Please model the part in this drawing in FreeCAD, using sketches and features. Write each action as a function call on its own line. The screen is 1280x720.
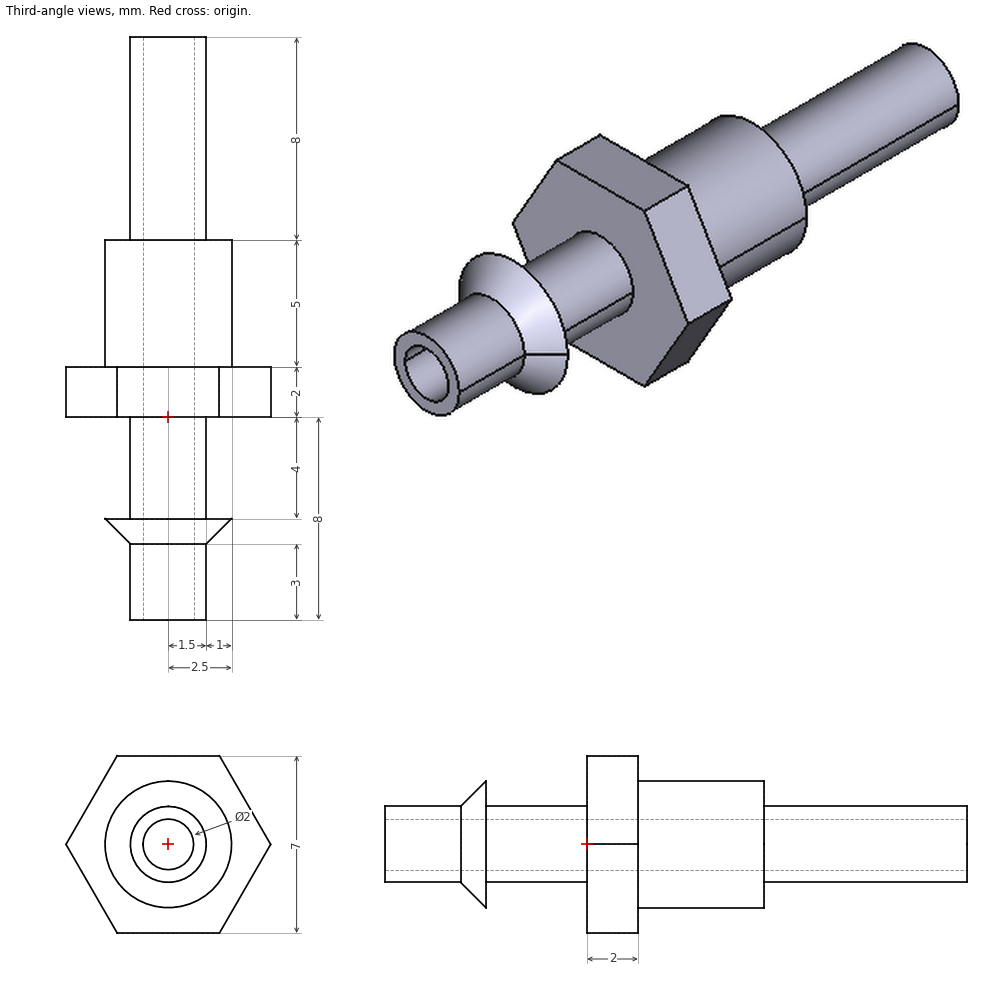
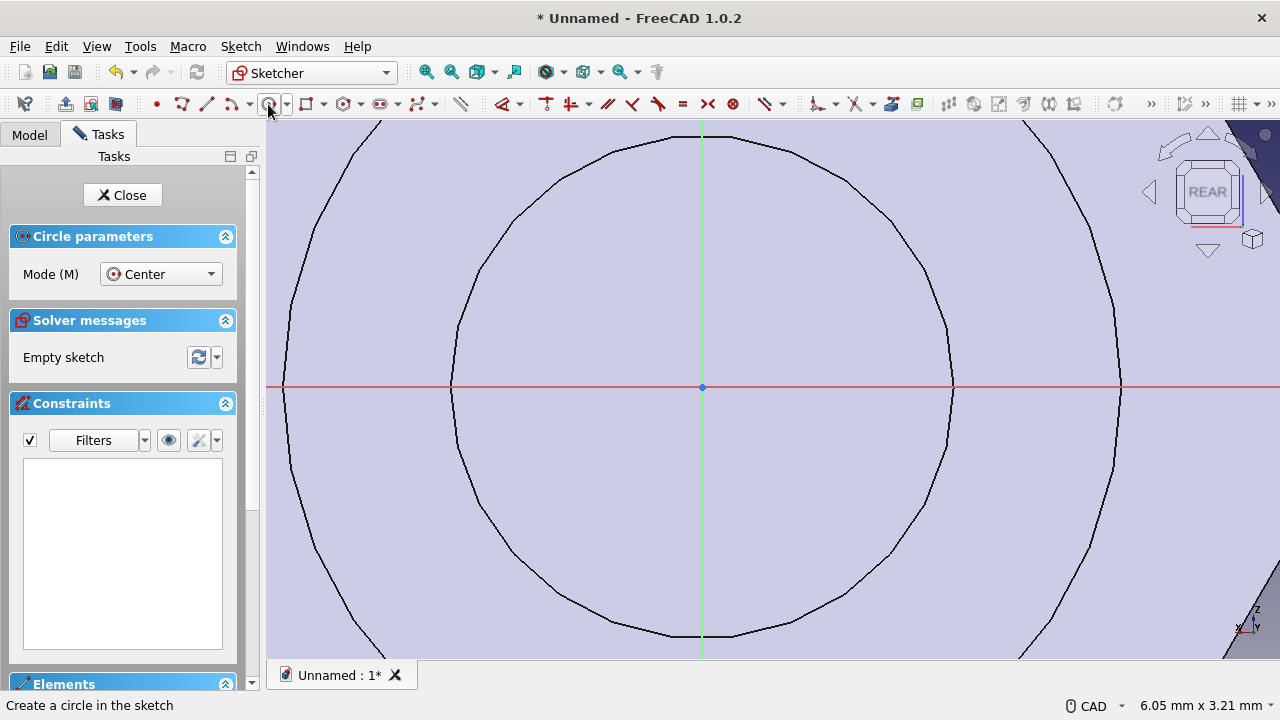
click(702, 387)
move(821, 269)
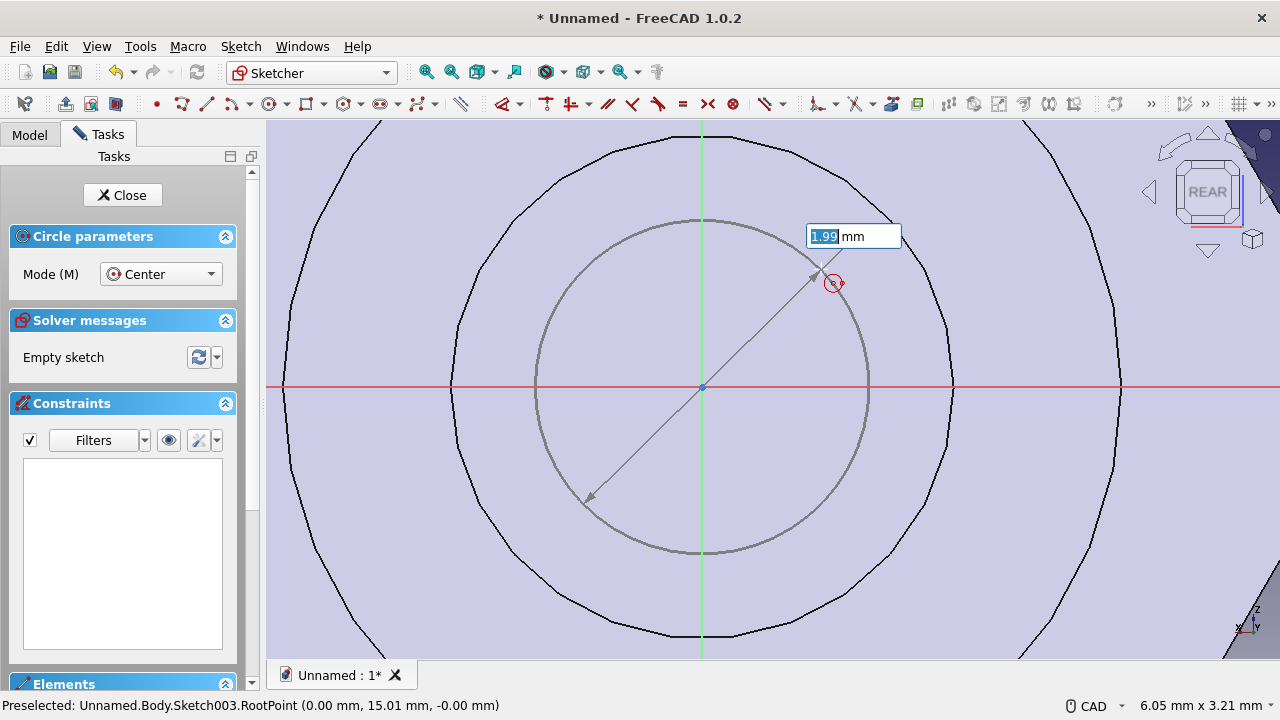
text(2)
key(Return)
key(Escape)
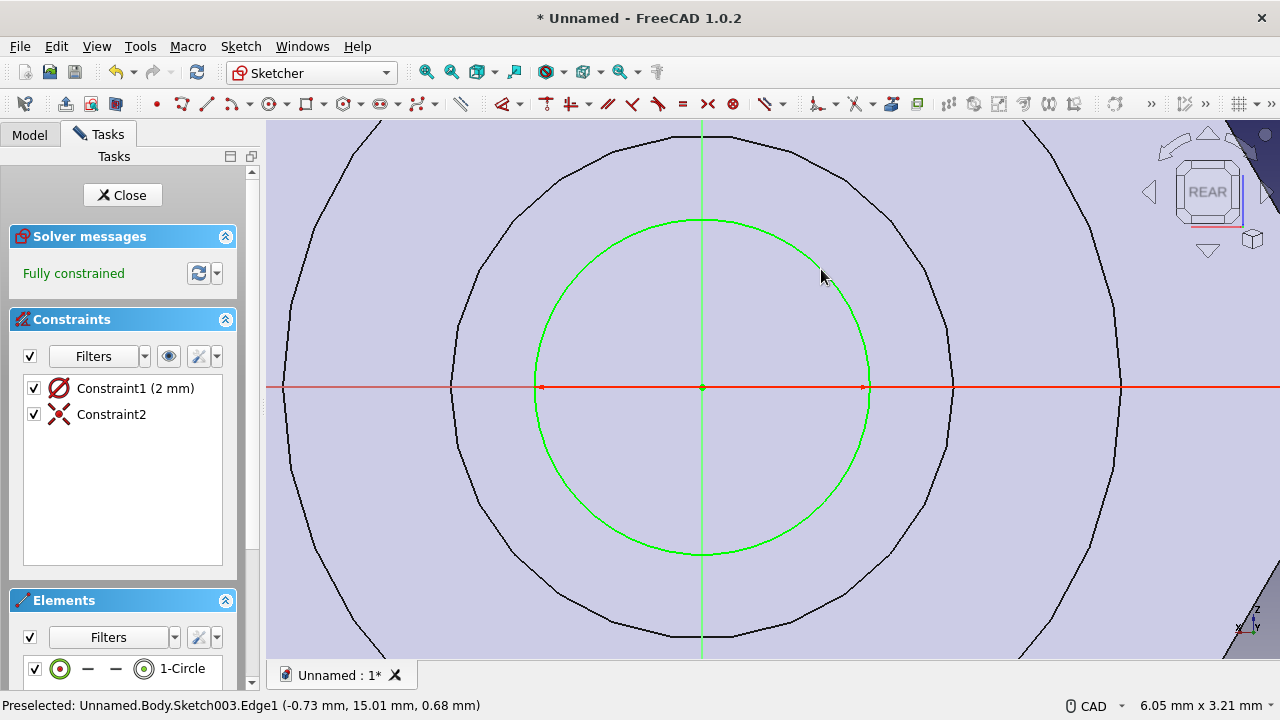
click(123, 195)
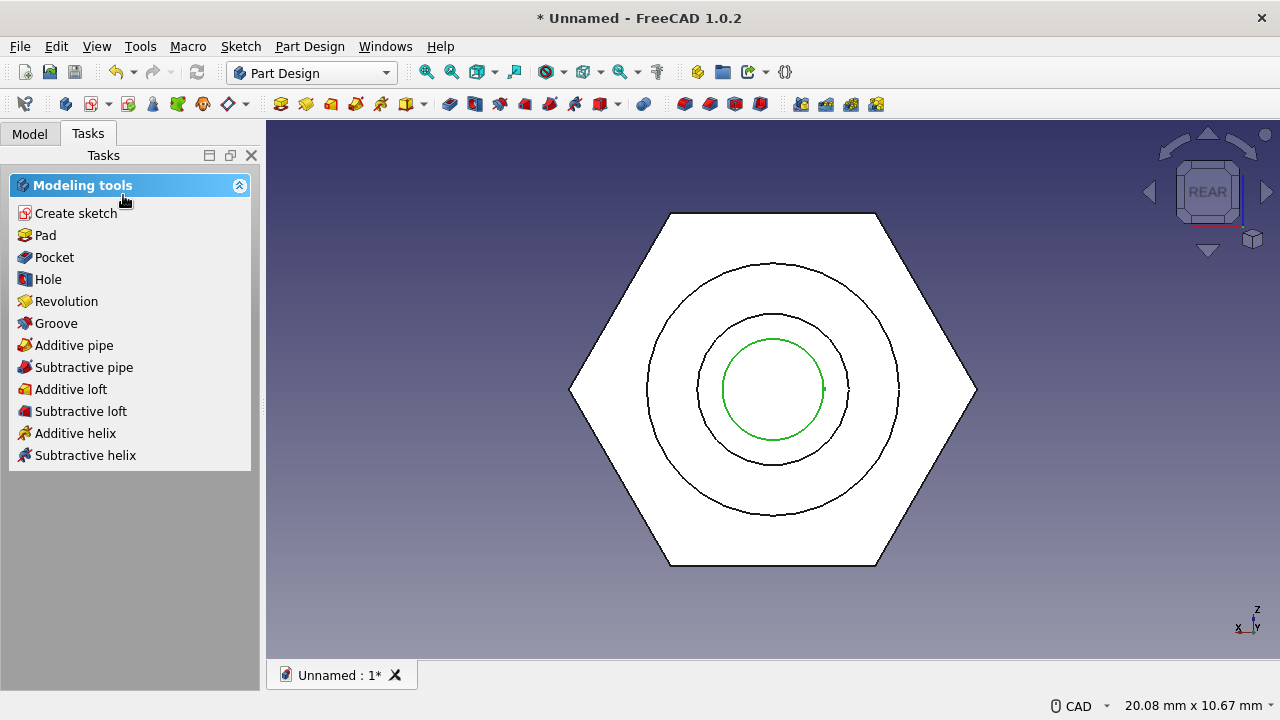
click(450, 104)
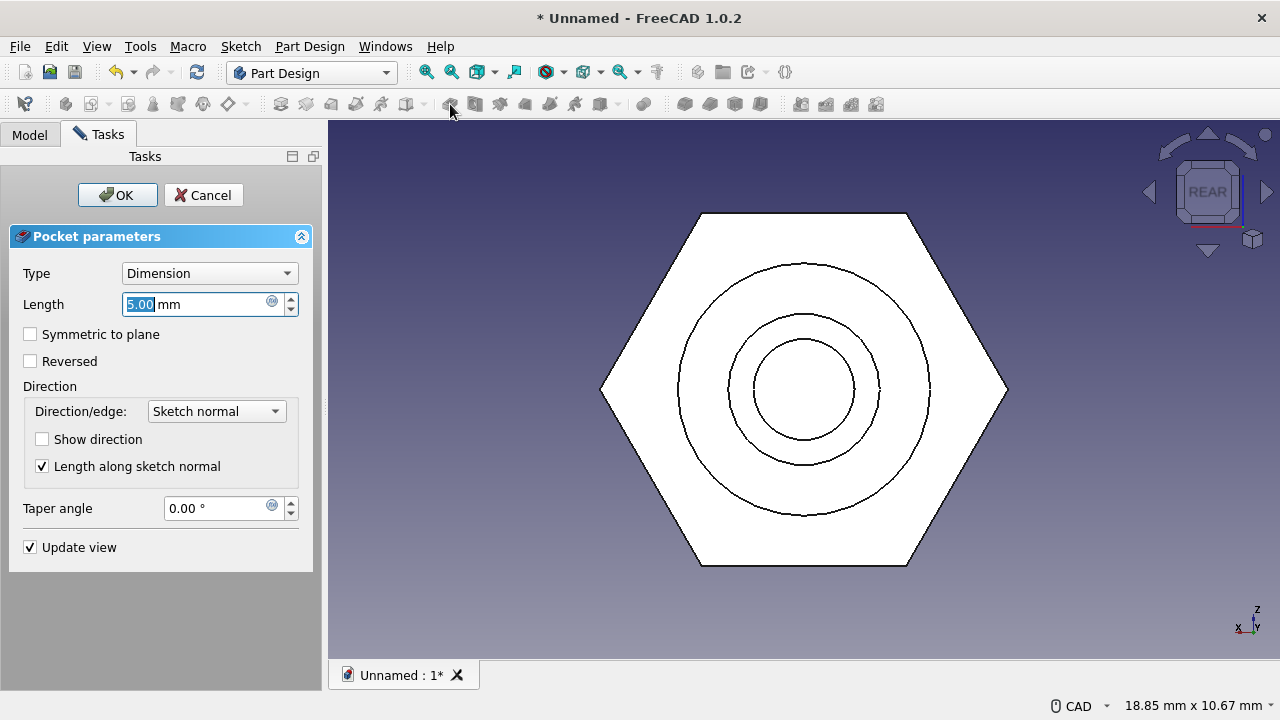
click(210, 274)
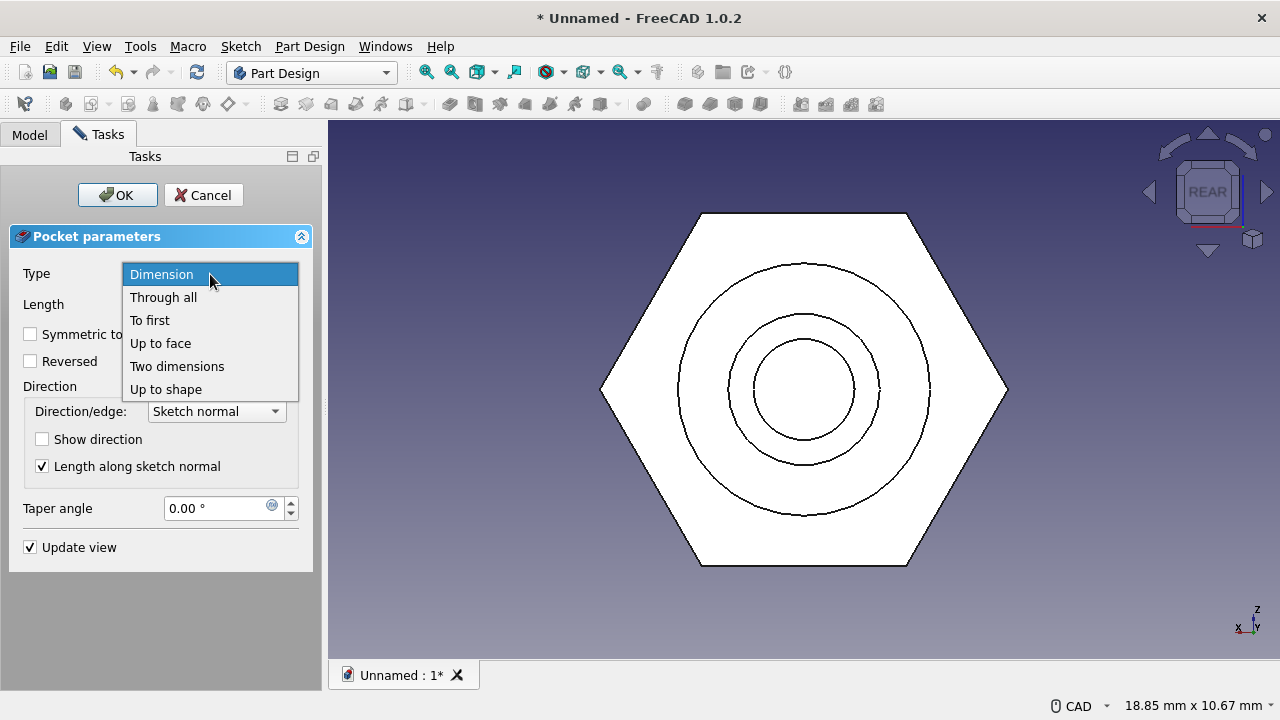
click(208, 298)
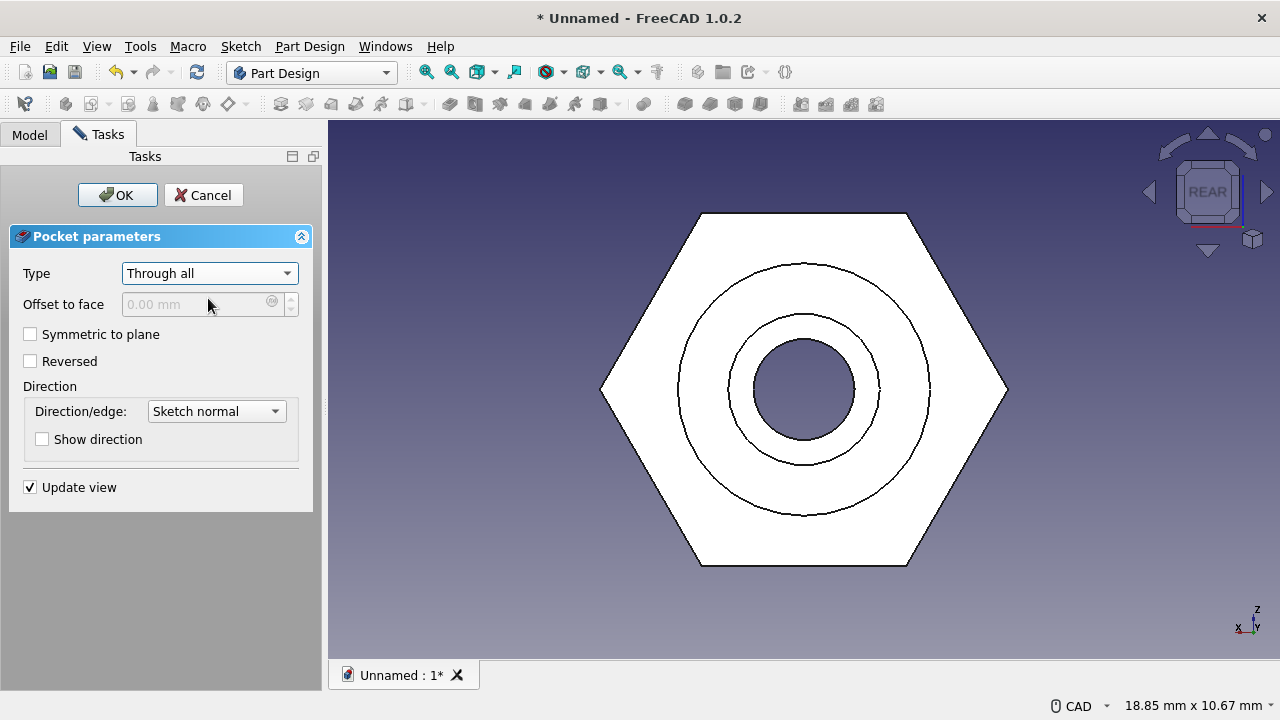
click(118, 195)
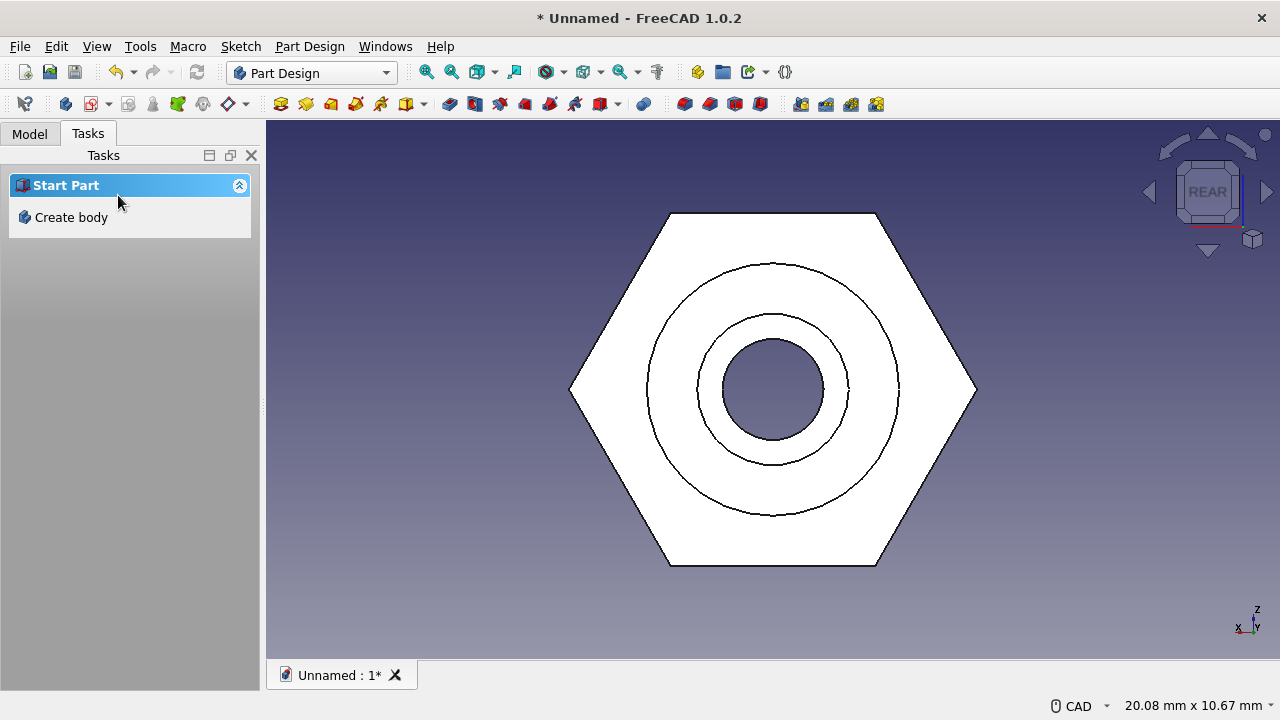
key(0)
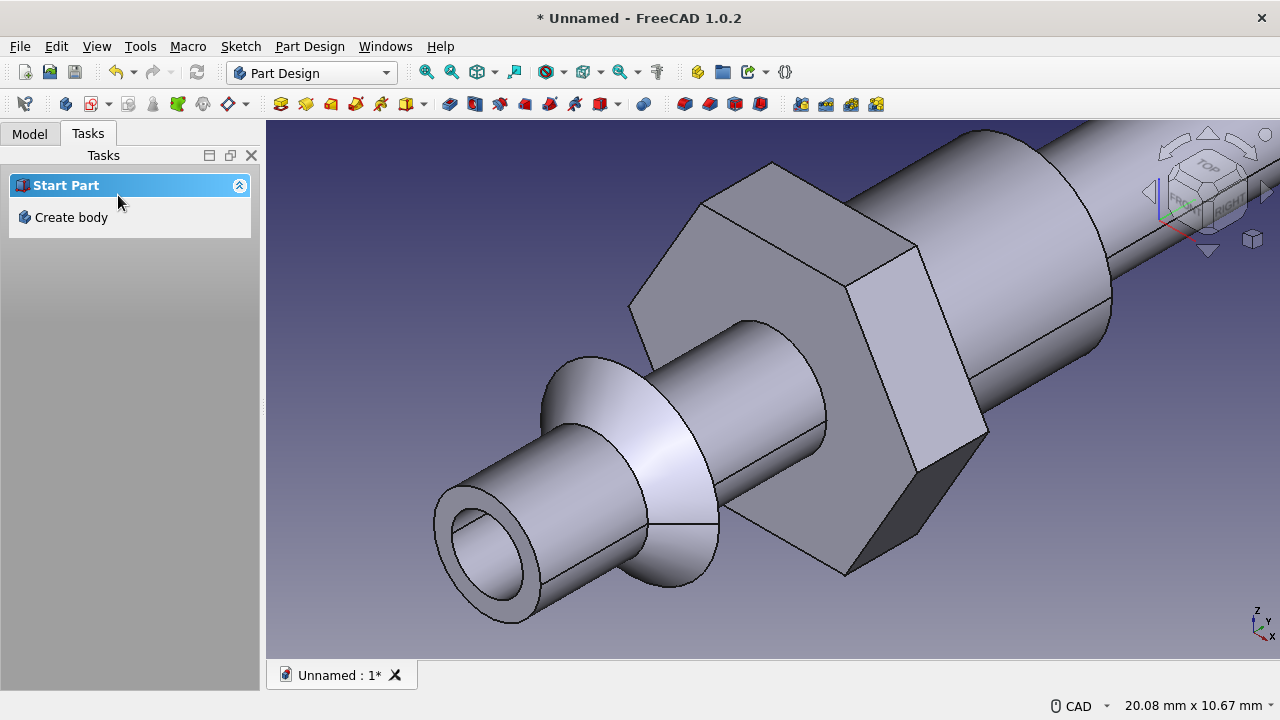
click(427, 72)